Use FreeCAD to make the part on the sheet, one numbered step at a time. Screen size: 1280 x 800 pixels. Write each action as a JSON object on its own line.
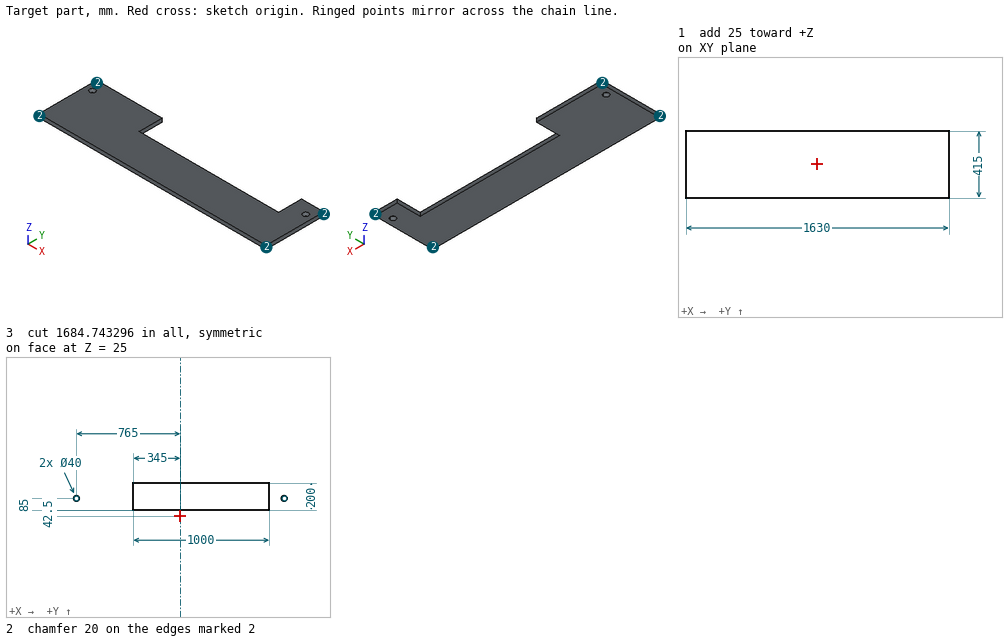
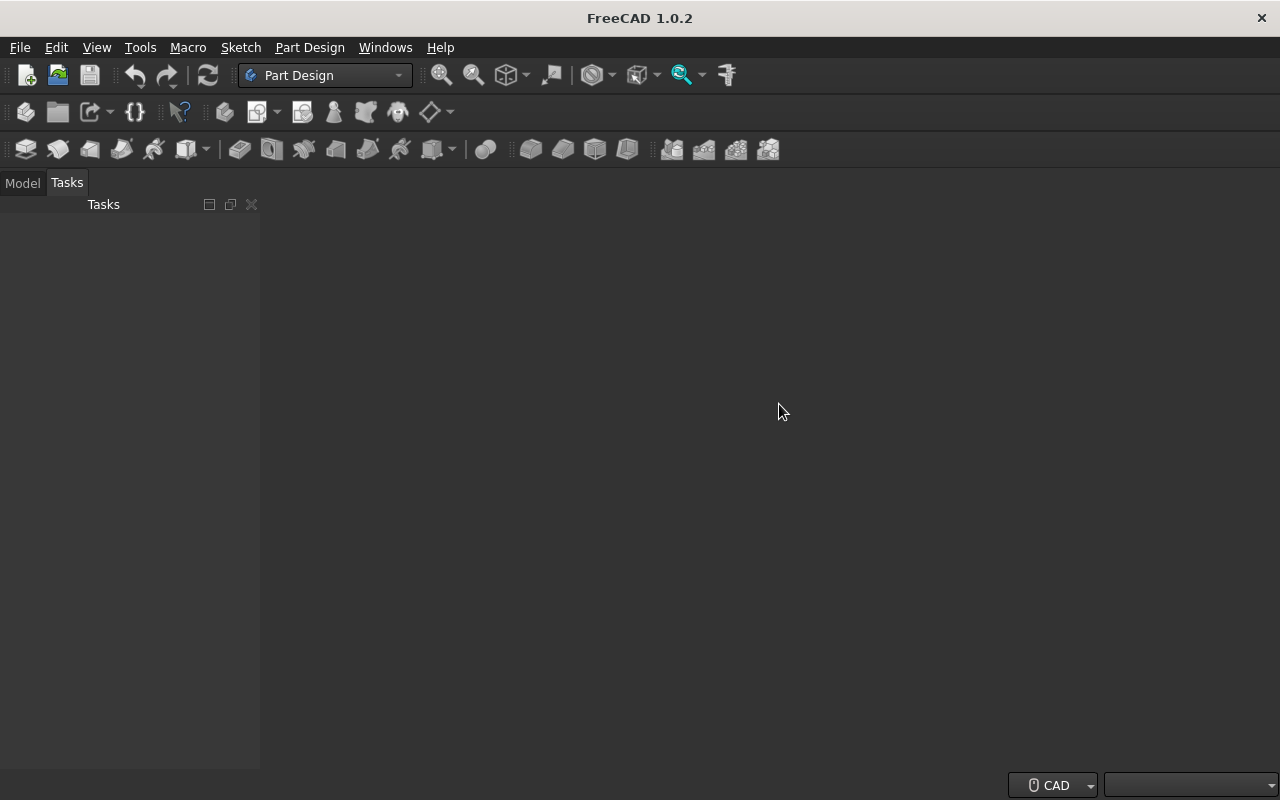
{"action": "left_click", "coordinate": [26, 76]}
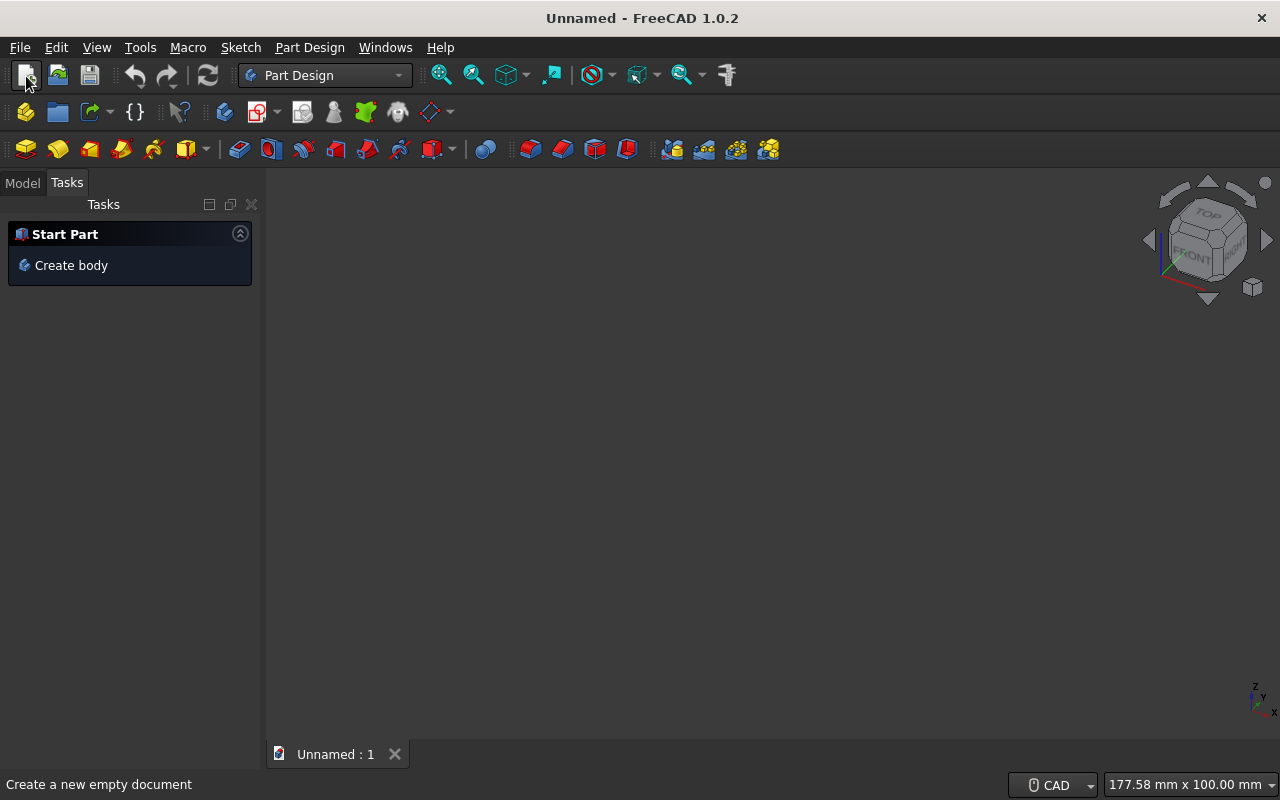
{"action": "left_click", "coordinate": [258, 112]}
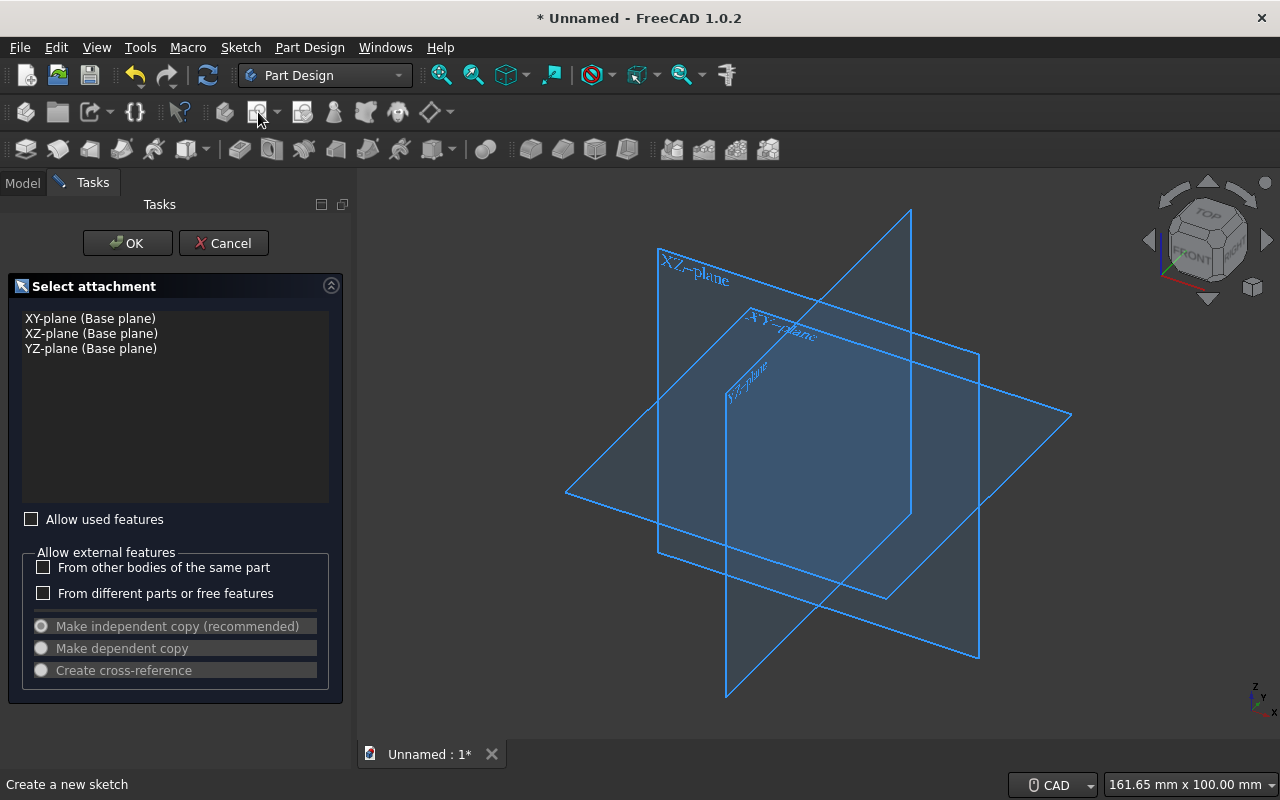
{"action": "left_click", "coordinate": [82, 318]}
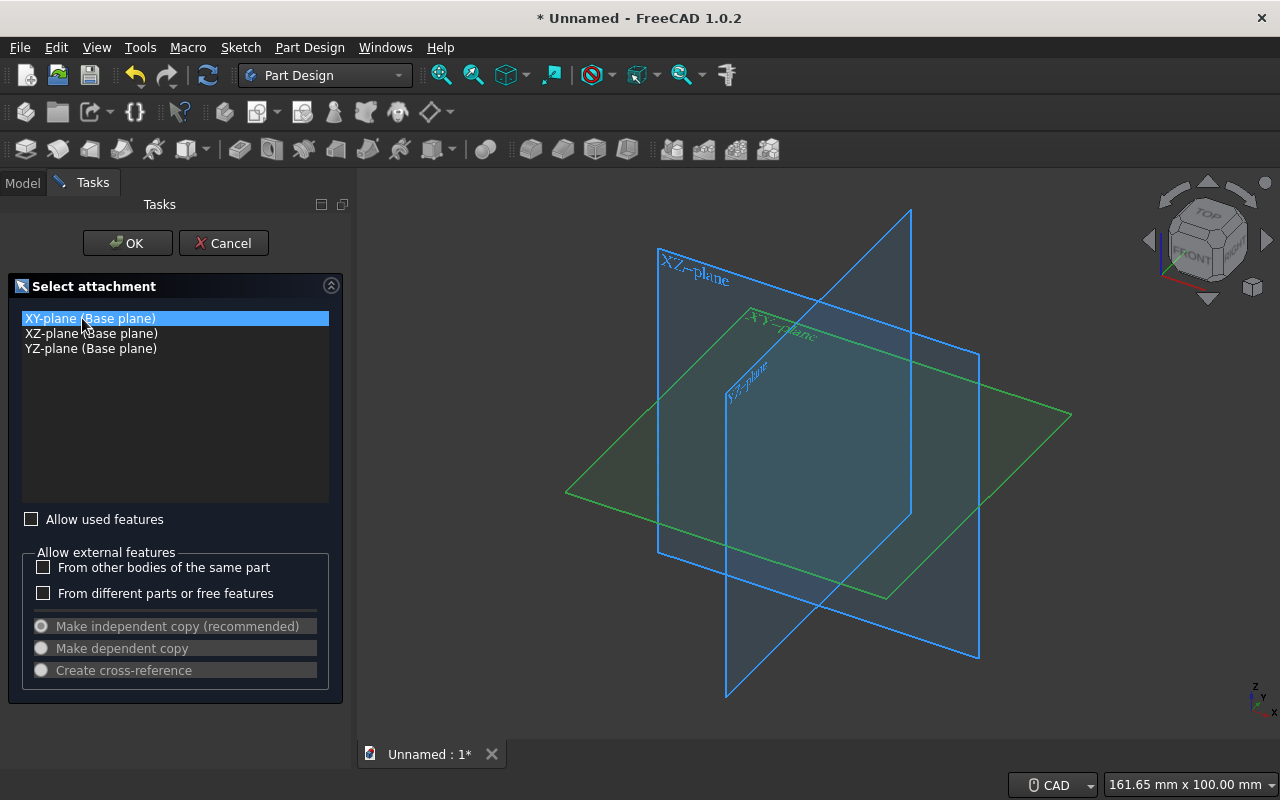
{"action": "left_click", "coordinate": [128, 243]}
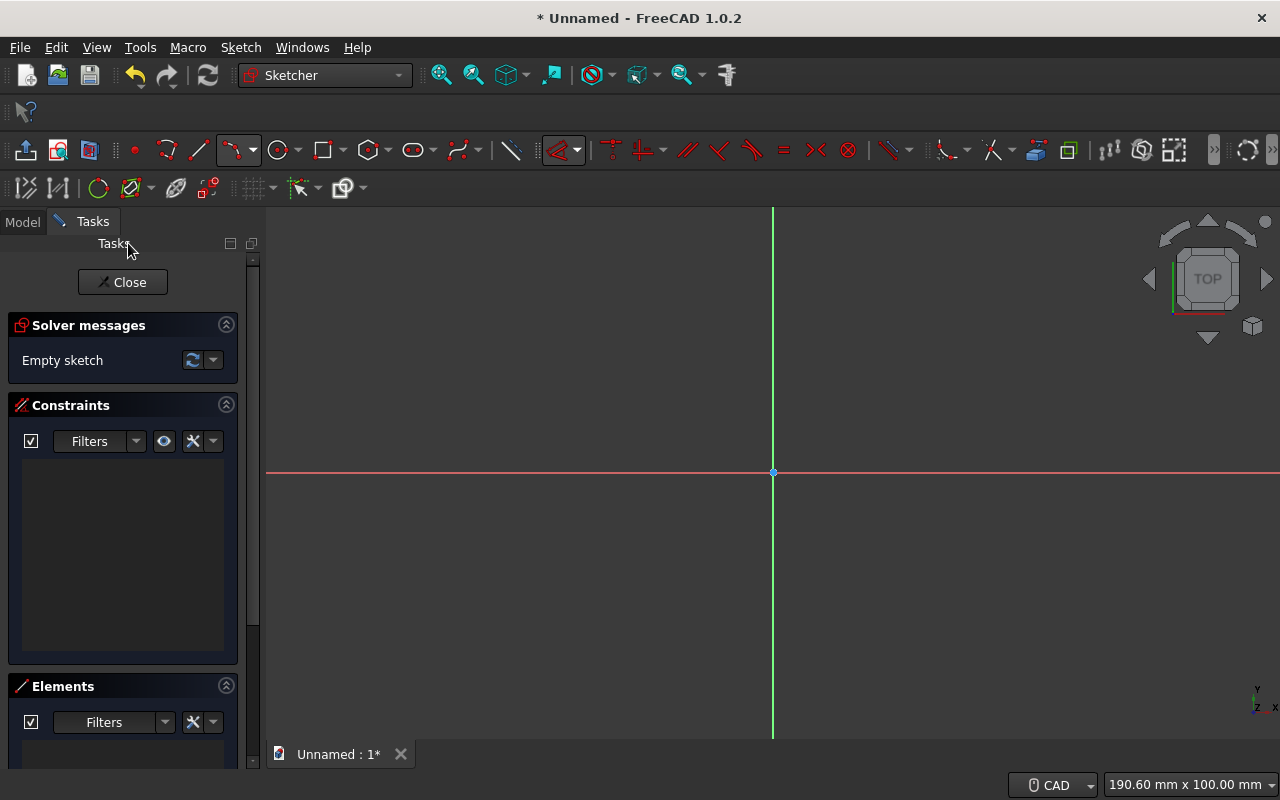
{"action": "scroll", "coordinate": [700, 473], "scroll_direction": "down", "scroll_amount": 14}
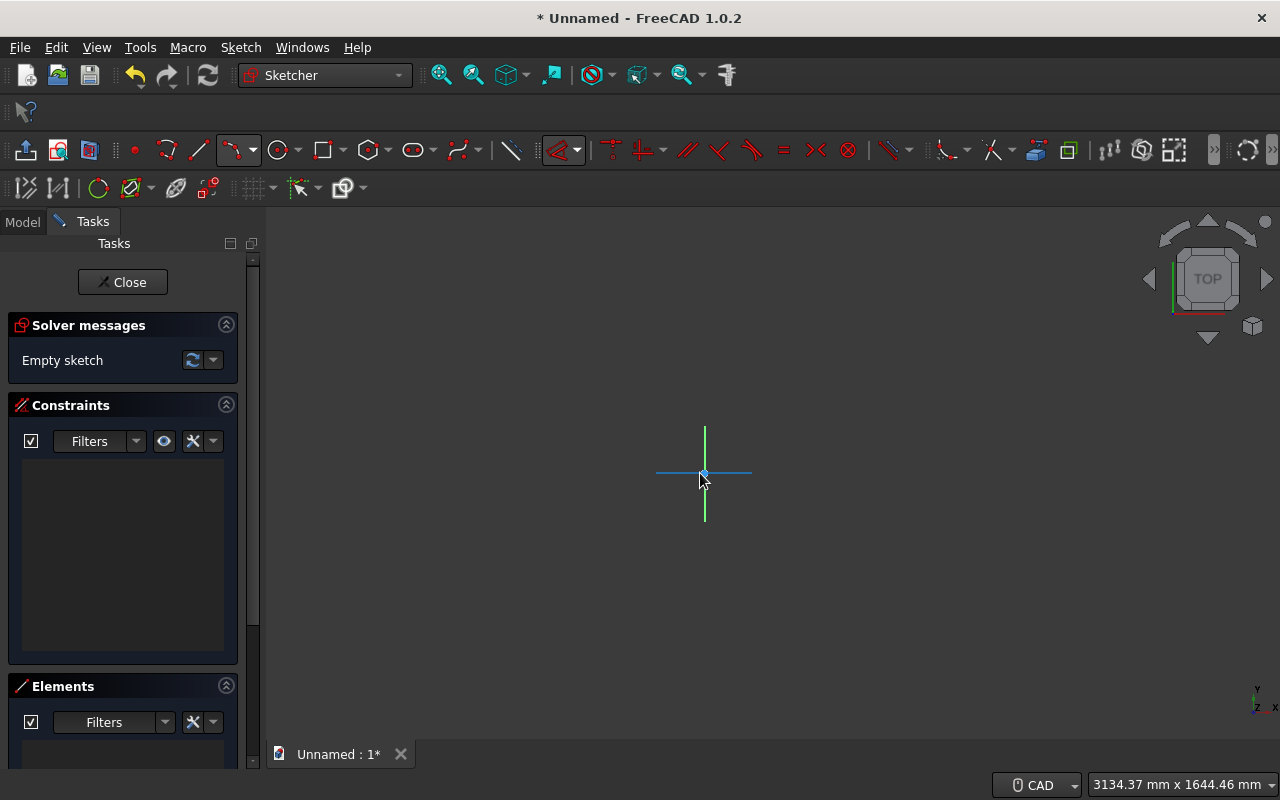
{"action": "left_click", "coordinate": [346, 150]}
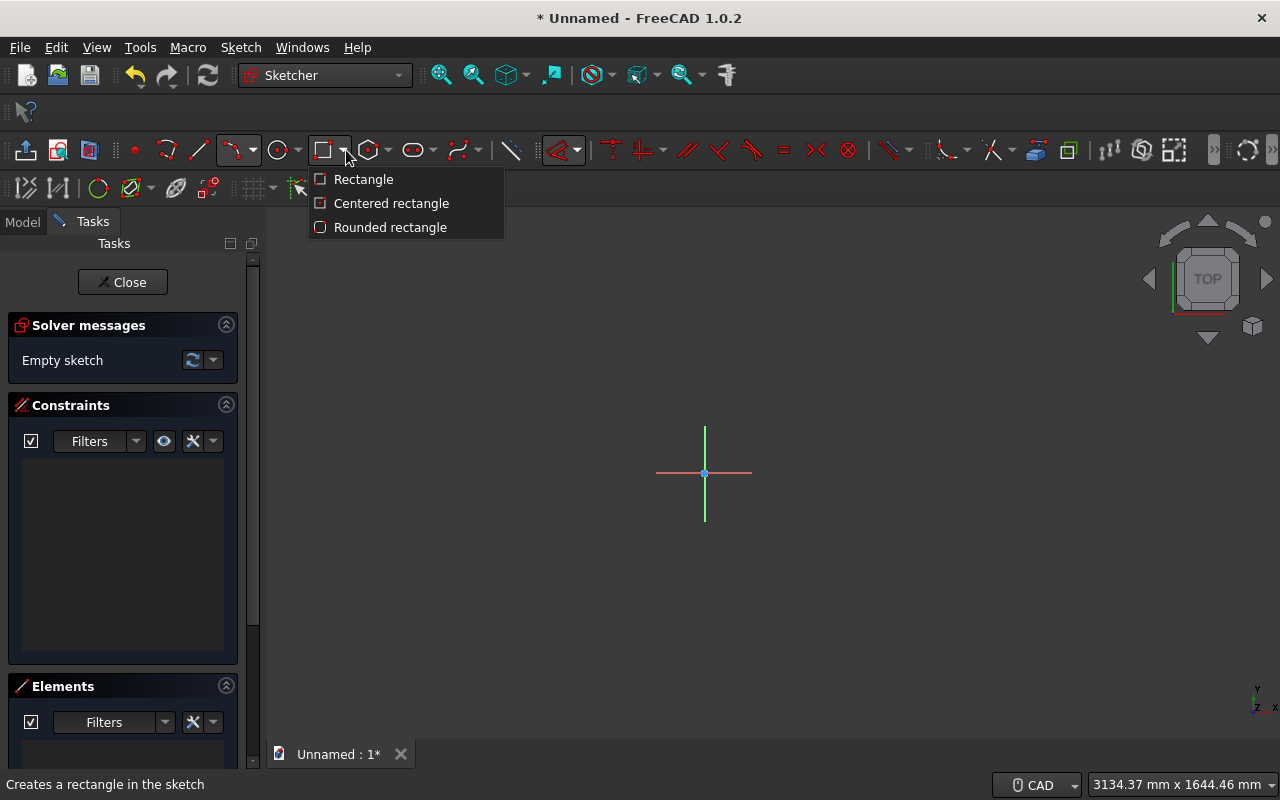
{"action": "left_click", "coordinate": [406, 203]}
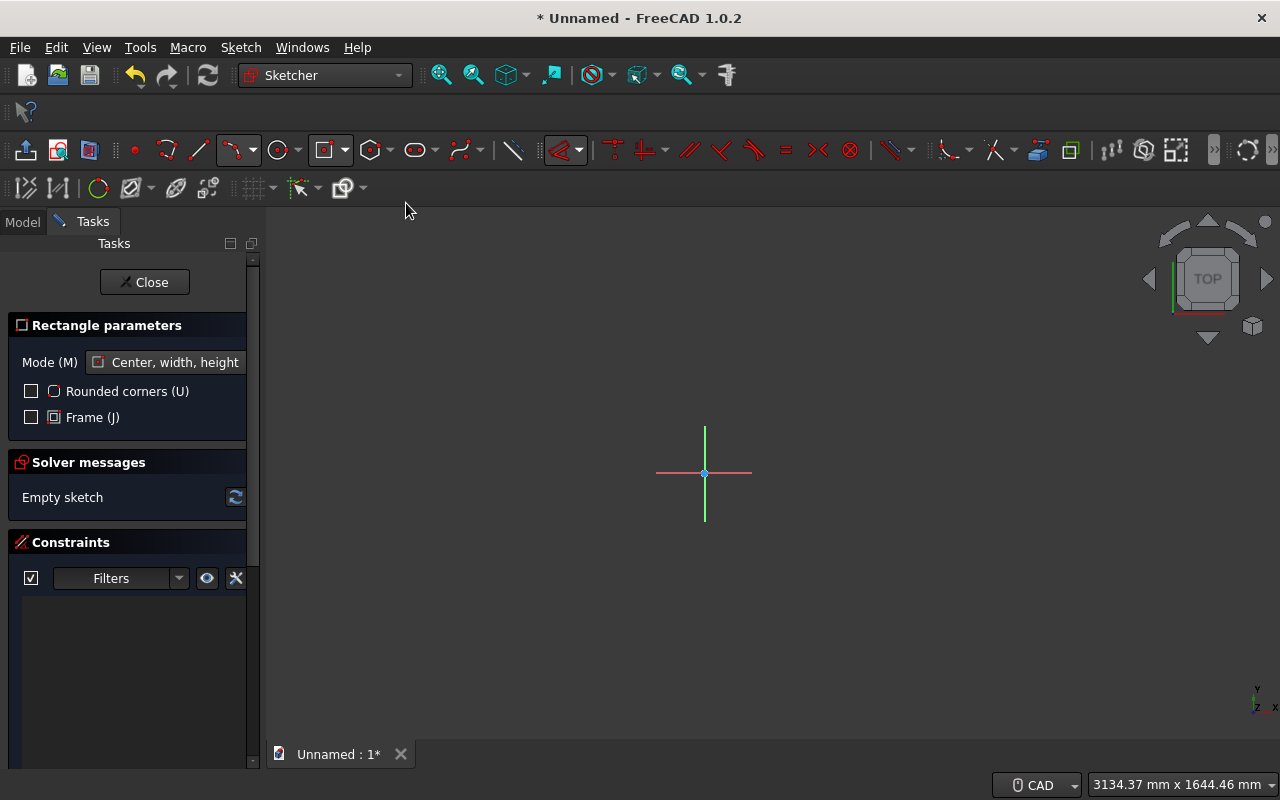
{"action": "left_click", "coordinate": [705, 473]}
{"action": "mouse_move", "coordinate": [969, 406]}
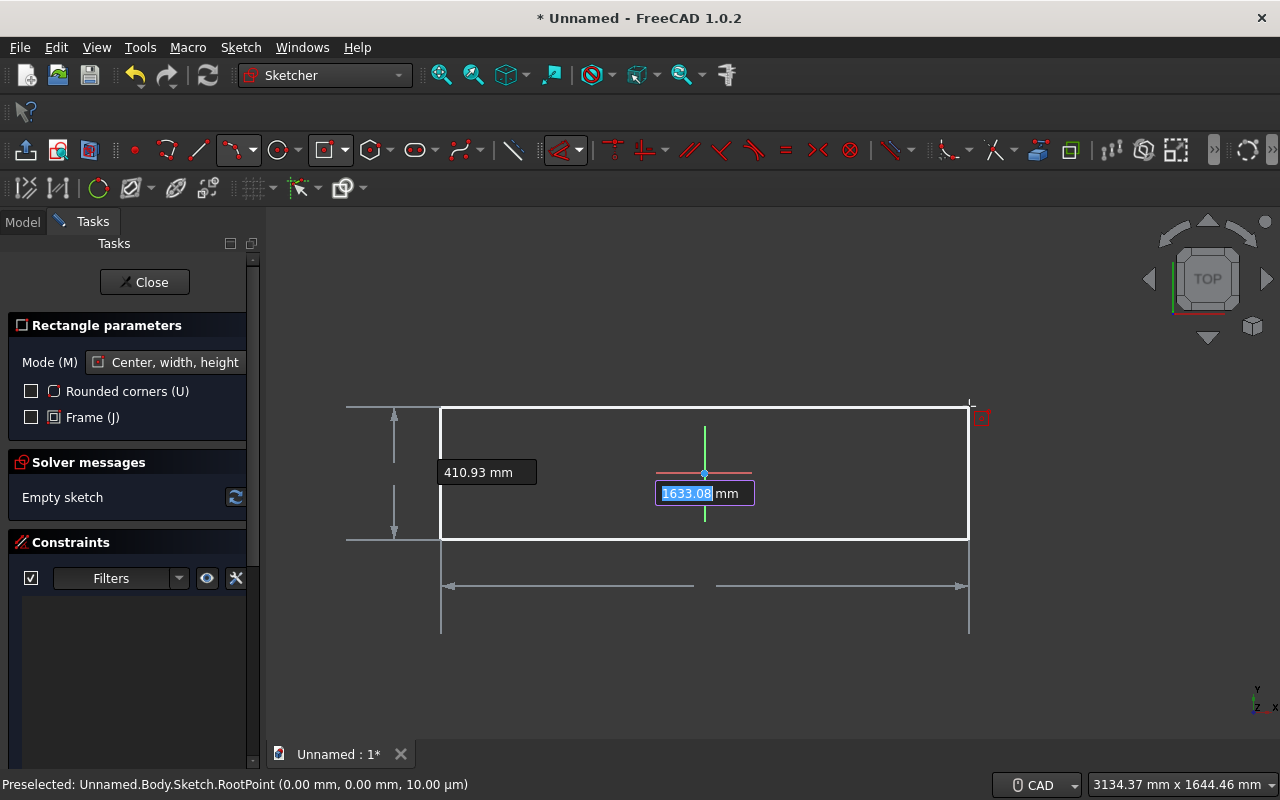
{"action": "type", "text": "1630"}
{"action": "key", "text": "Tab"}
{"action": "type", "text": "415"}
{"action": "key", "text": "Return"}
{"action": "key", "text": "Escape"}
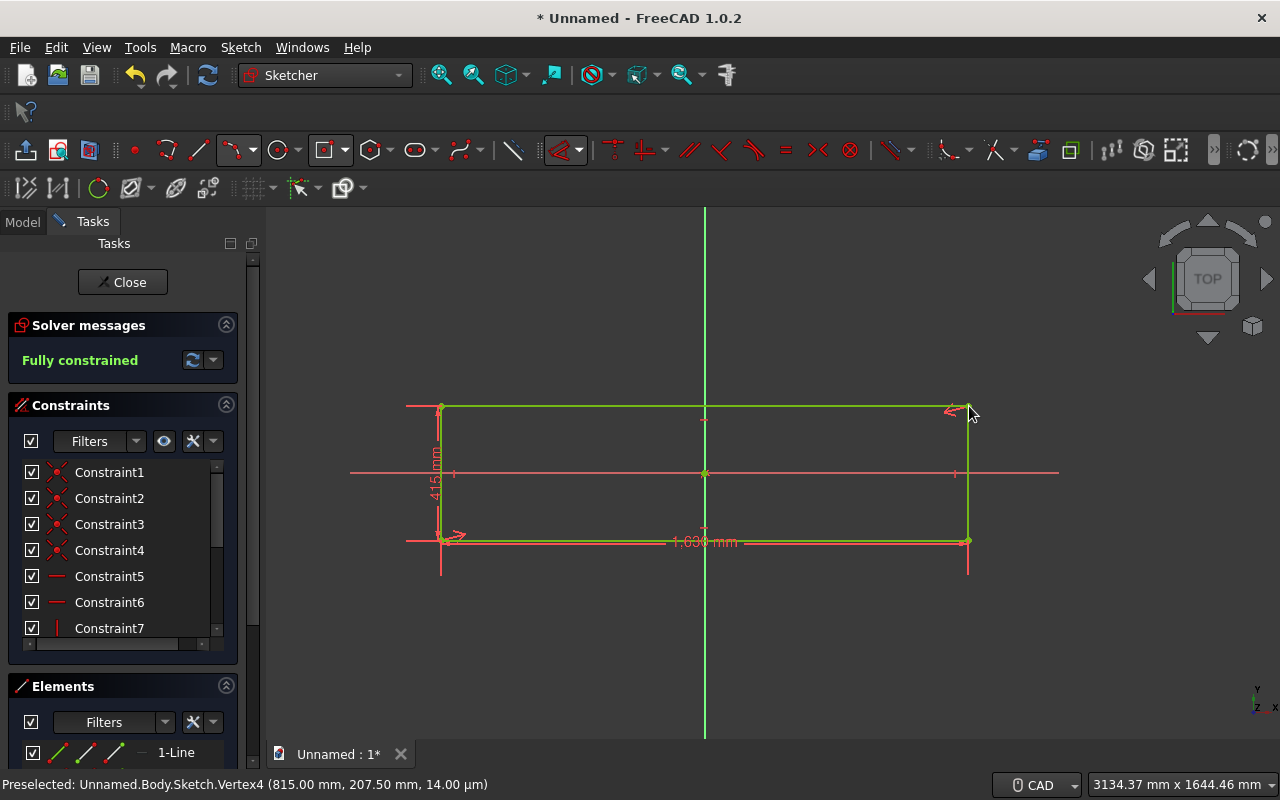
{"action": "left_click", "coordinate": [123, 282]}